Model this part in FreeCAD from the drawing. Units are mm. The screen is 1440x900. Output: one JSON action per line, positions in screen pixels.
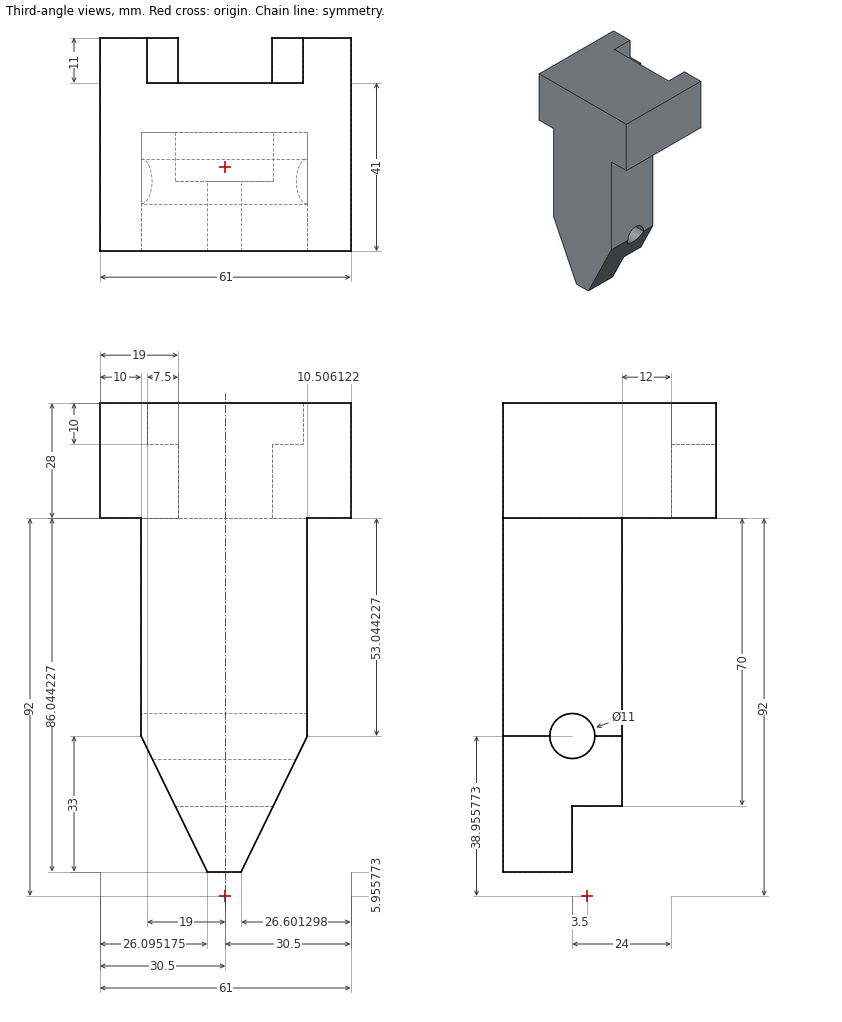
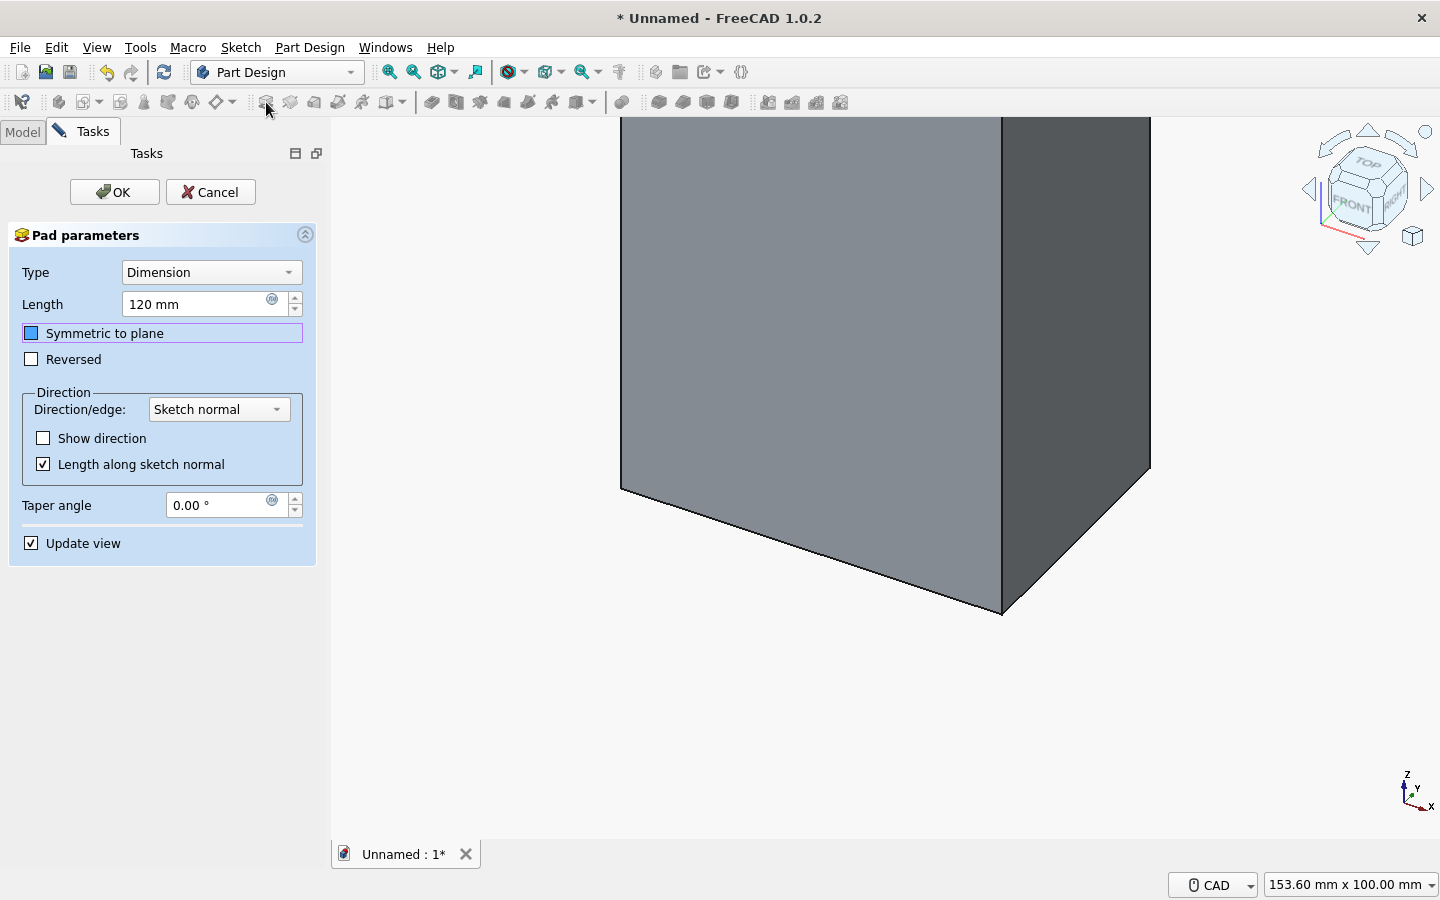
{"action": "left_click", "coordinate": [115, 192]}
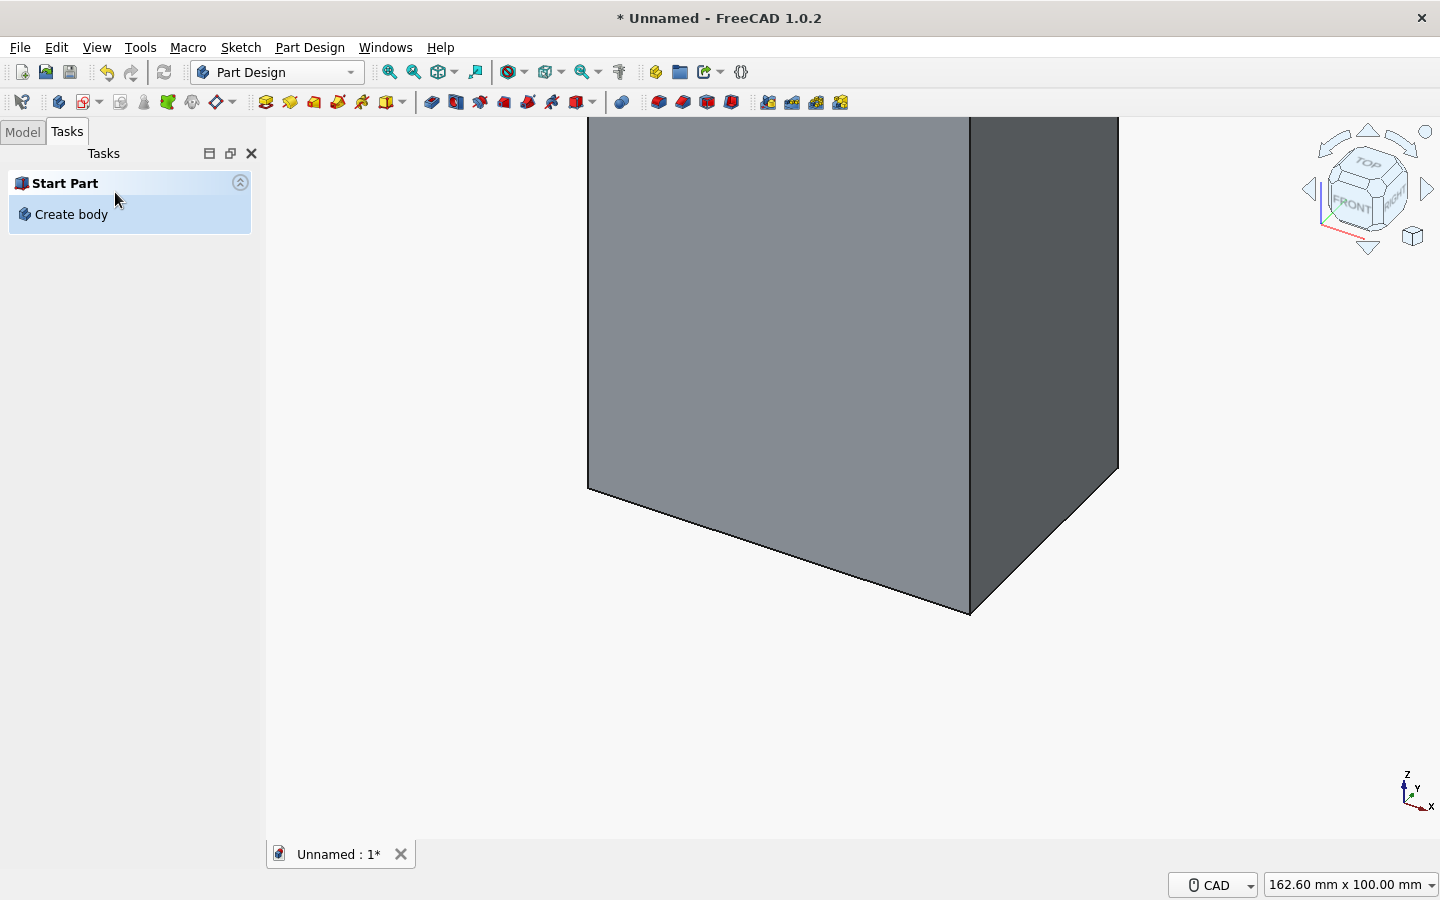
{"action": "left_click", "coordinate": [390, 72]}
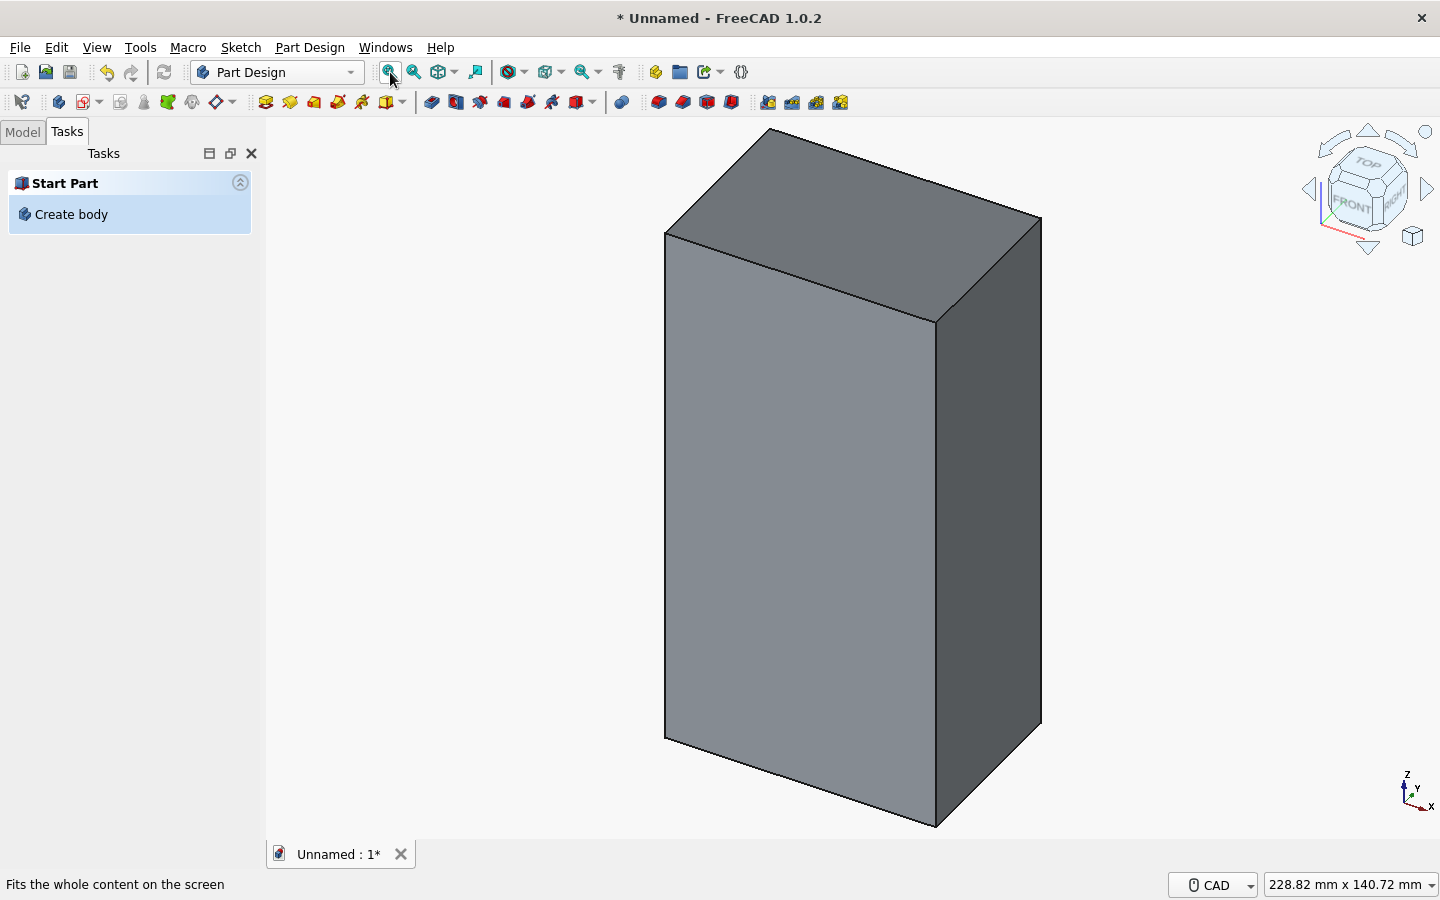
{"action": "left_click", "coordinate": [989, 378]}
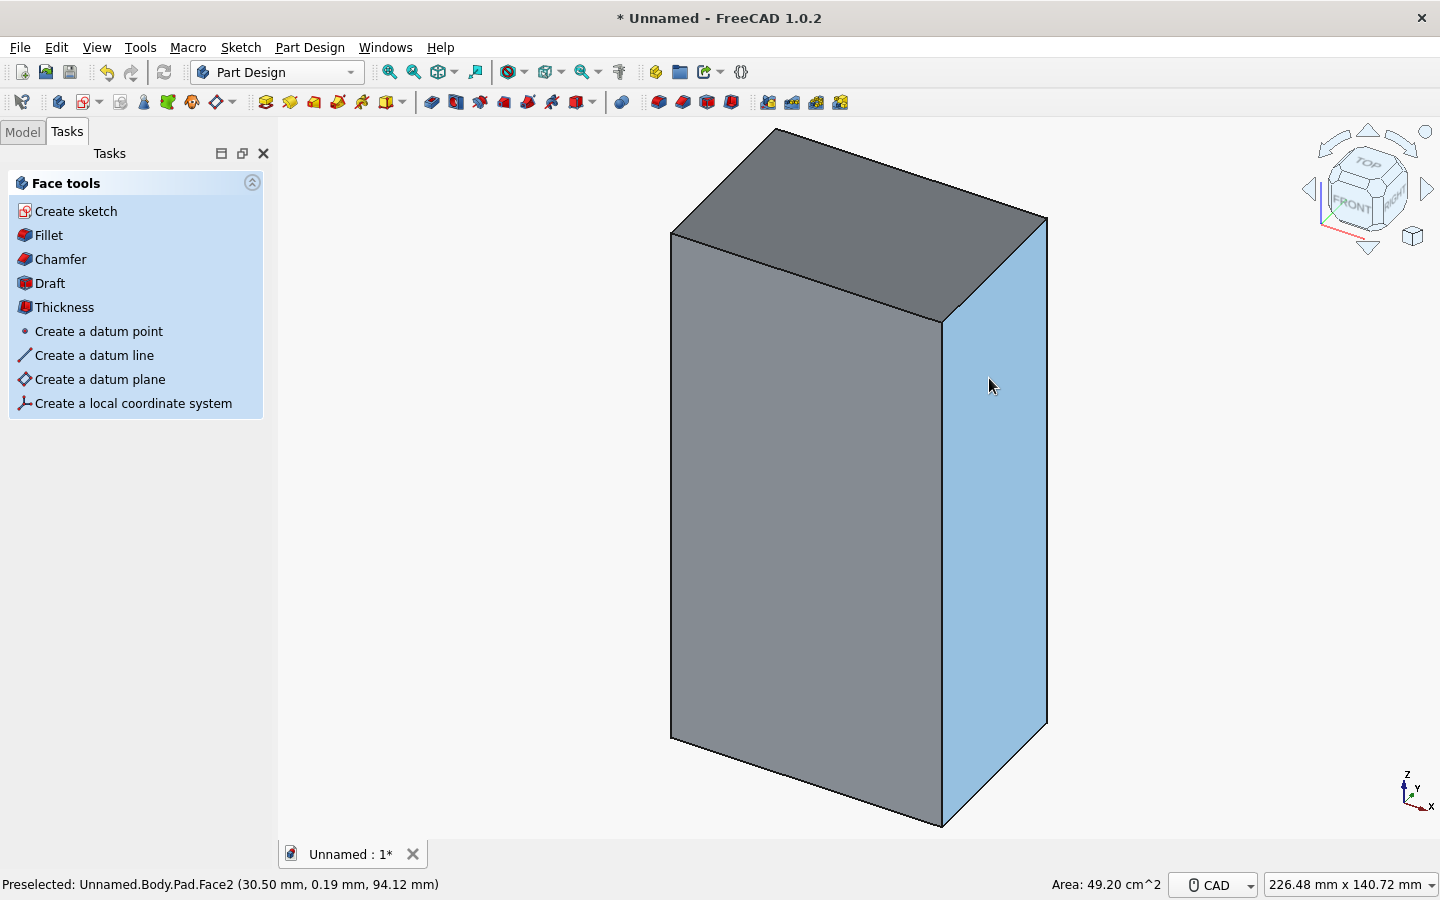
{"action": "left_click", "coordinate": [84, 102]}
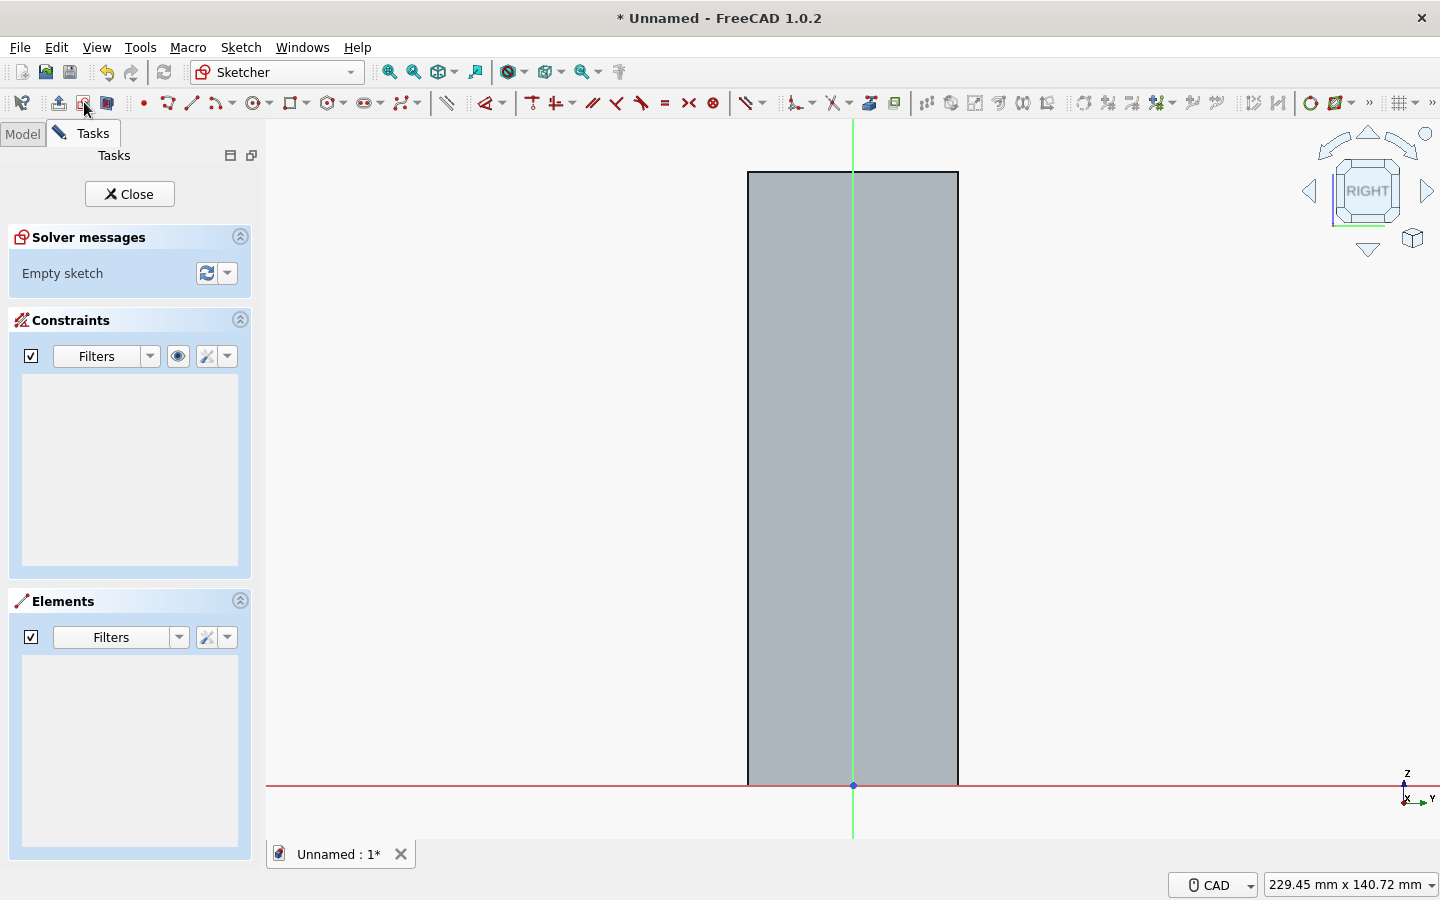
{"action": "left_click", "coordinate": [168, 104]}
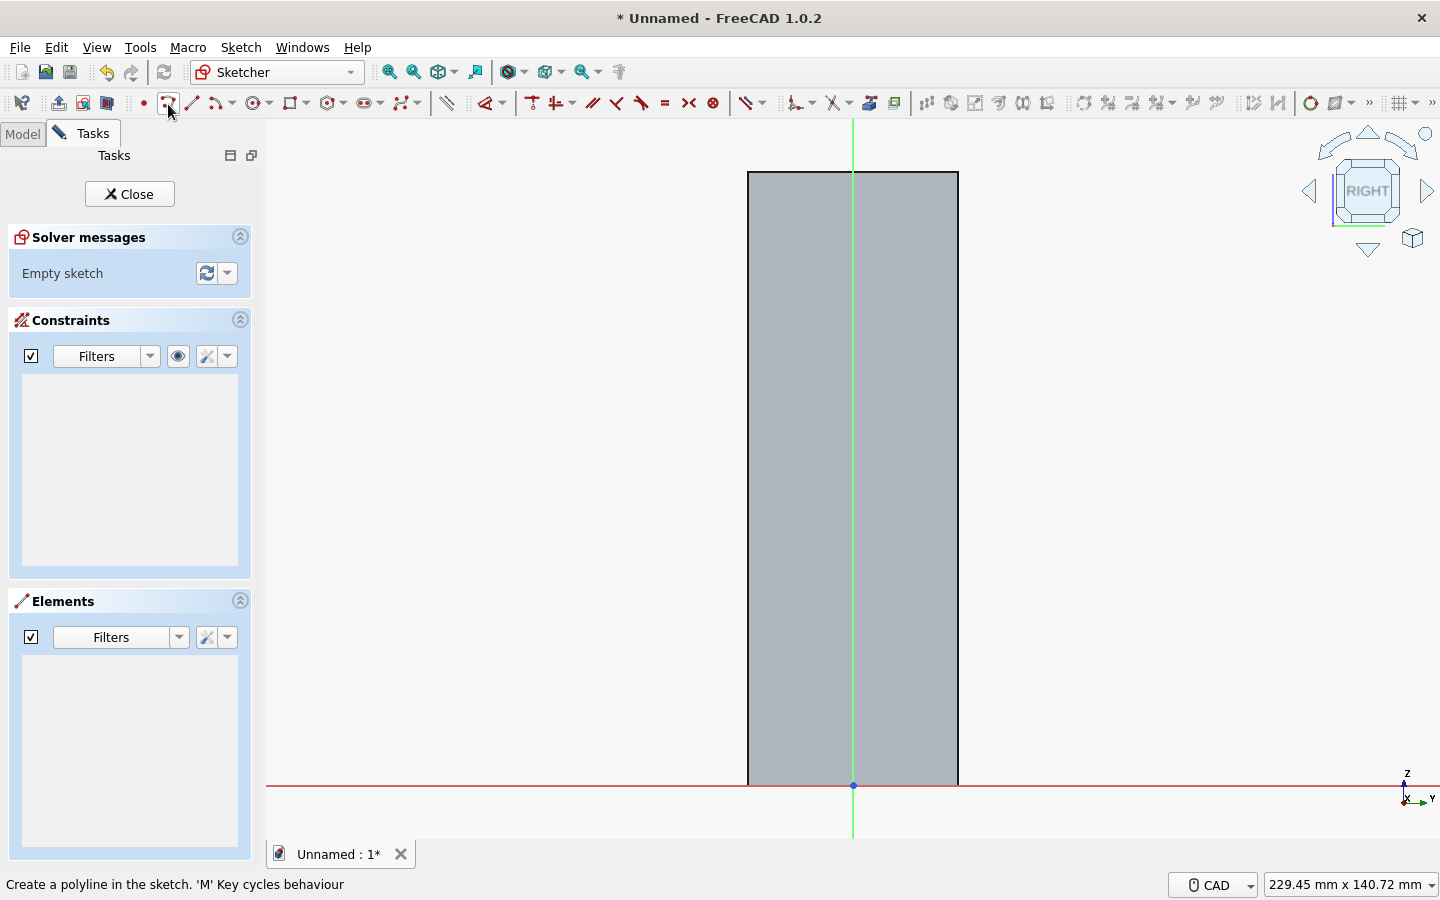
{"action": "left_click", "coordinate": [835, 786]}
{"action": "left_click", "coordinate": [958, 777]}
{"action": "left_click", "coordinate": [958, 315]}
{"action": "left_click", "coordinate": [896, 315]}
{"action": "left_click", "coordinate": [896, 673]}
{"action": "left_click", "coordinate": [835, 673]}
{"action": "left_click", "coordinate": [835, 786]}
{"action": "key", "text": "Escape"}
{"action": "key", "text": "Escape"}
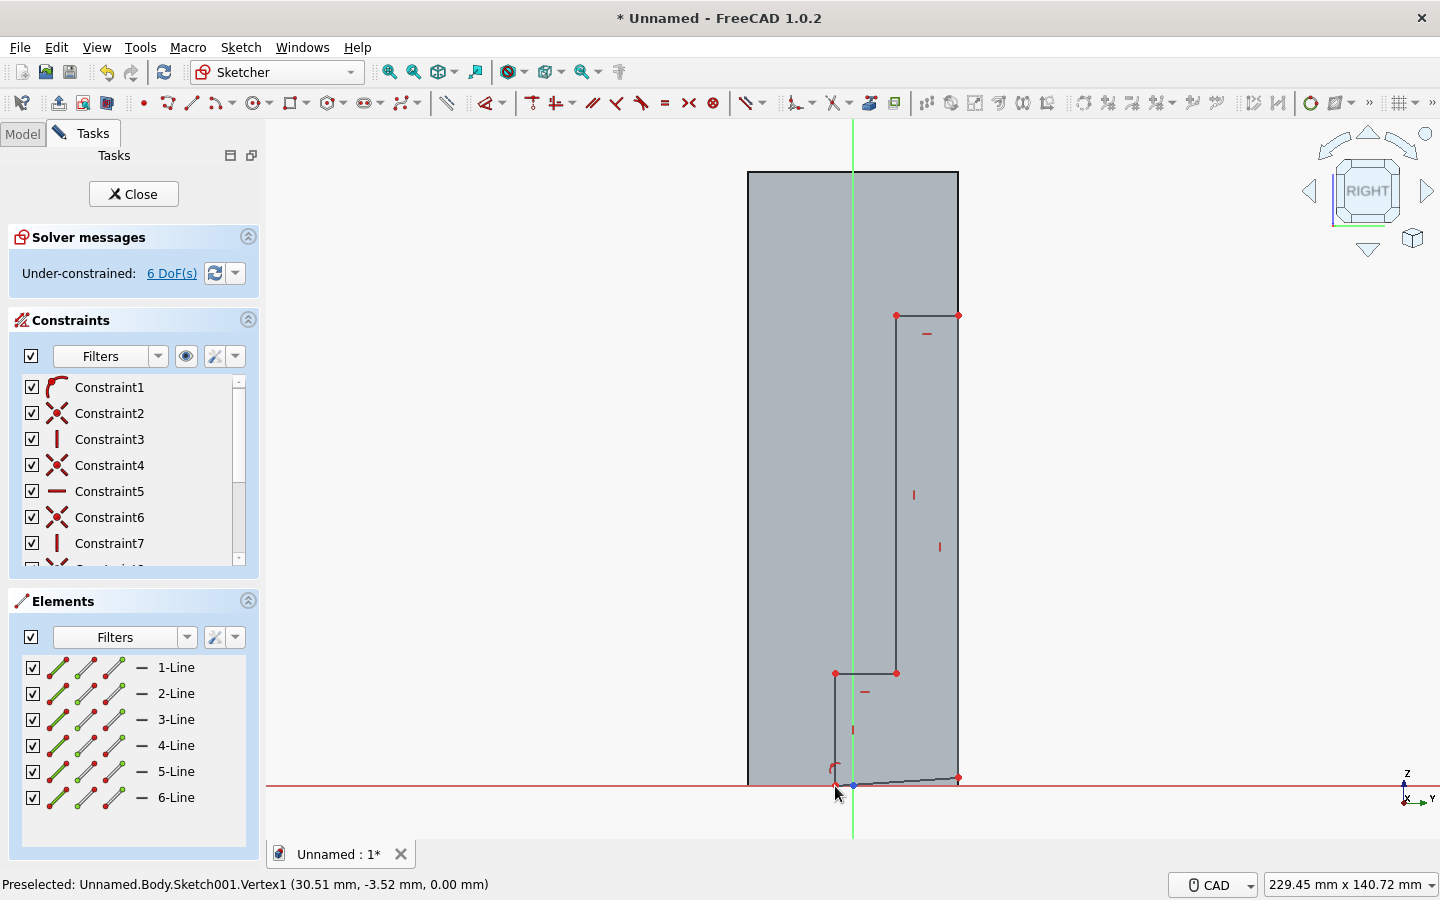
{"action": "left_click", "coordinate": [872, 784]}